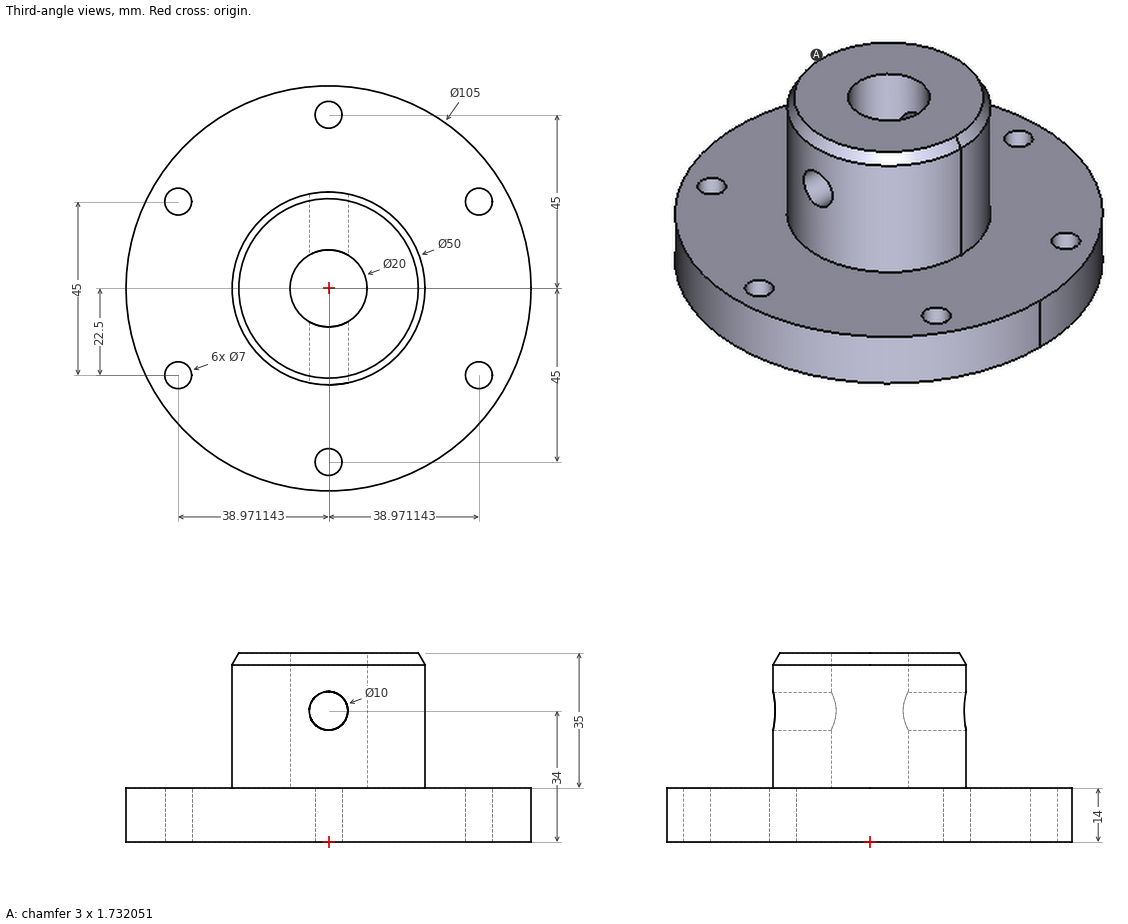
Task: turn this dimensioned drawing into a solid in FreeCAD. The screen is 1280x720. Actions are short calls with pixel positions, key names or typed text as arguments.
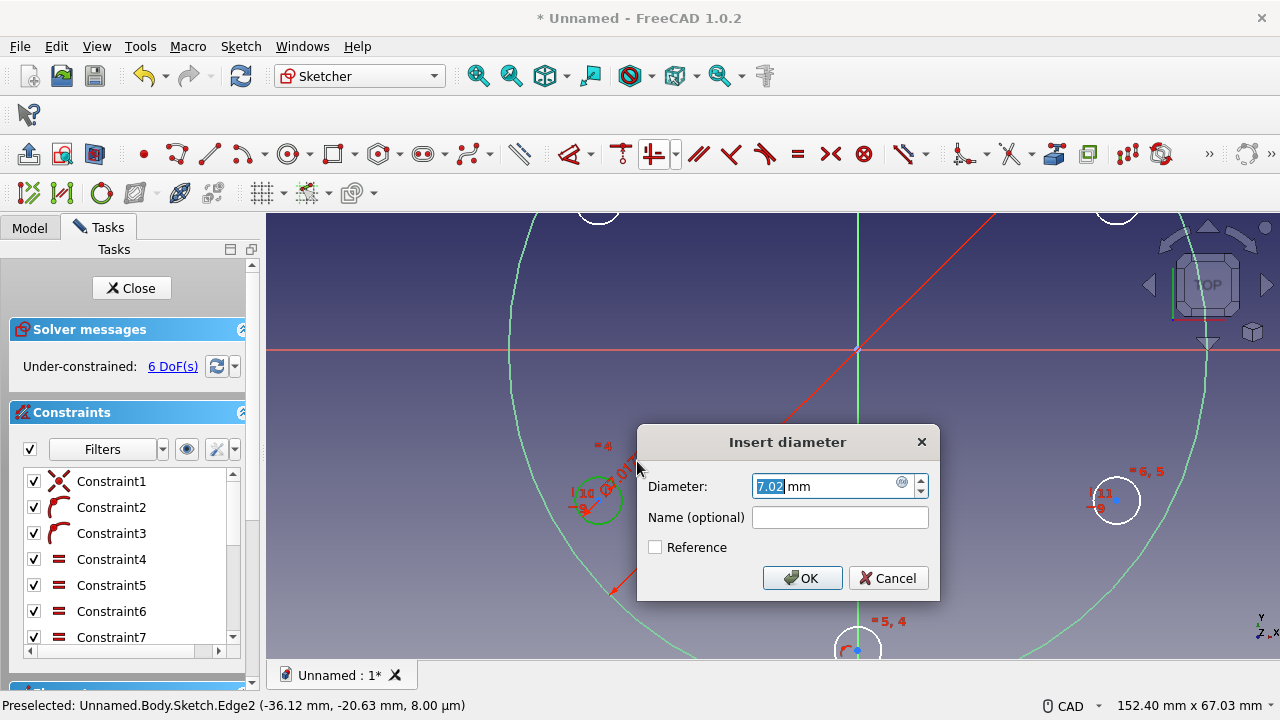
text(7)
key(Return)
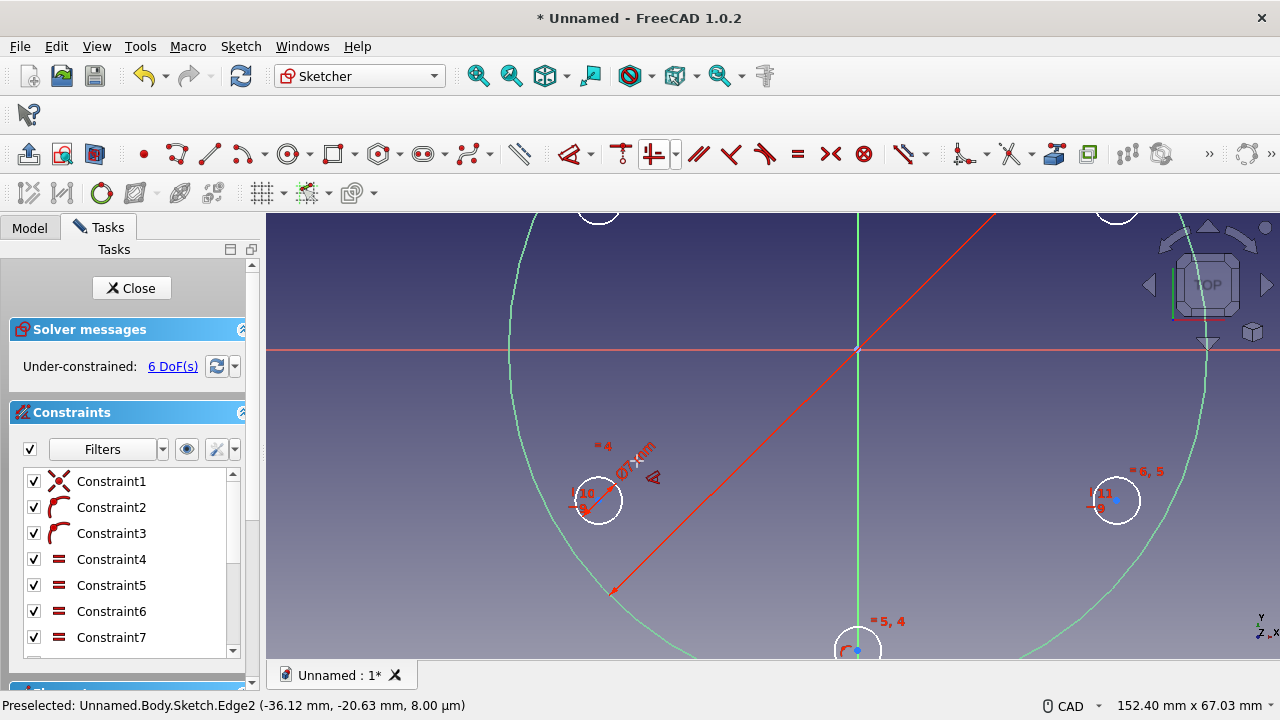
scroll(615, 486, down, 5)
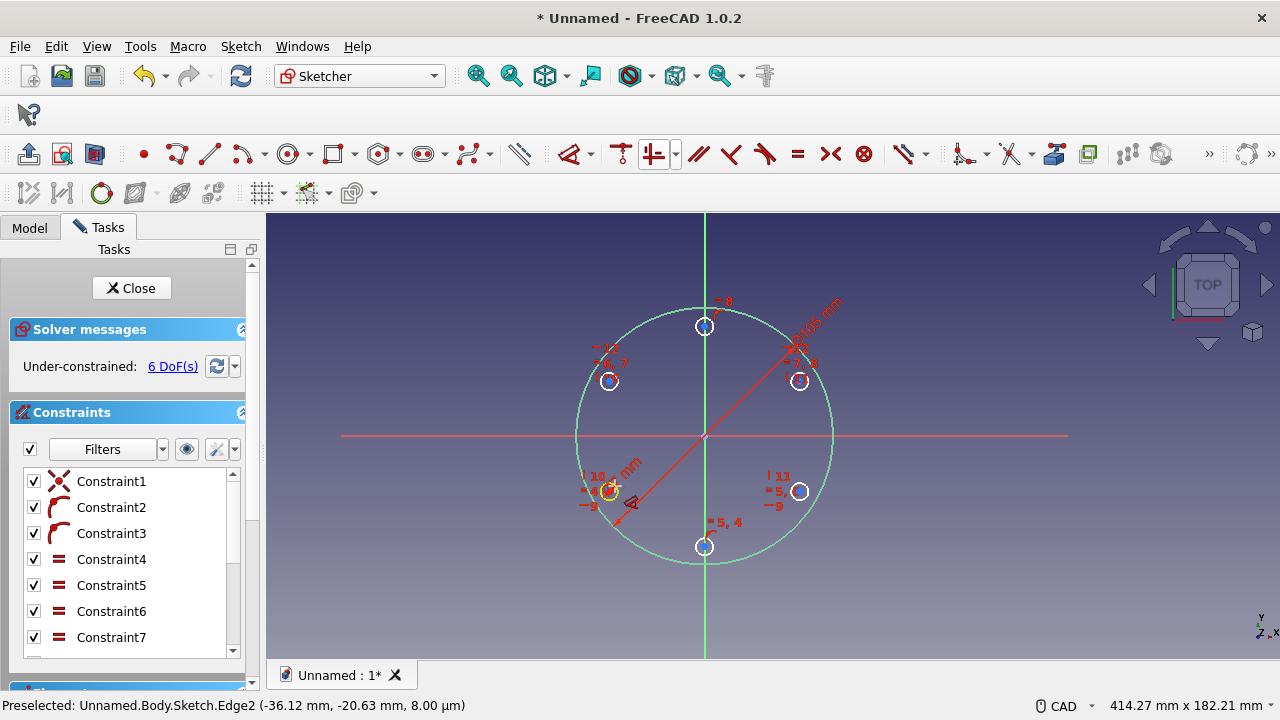
click(705, 547)
click(739, 492)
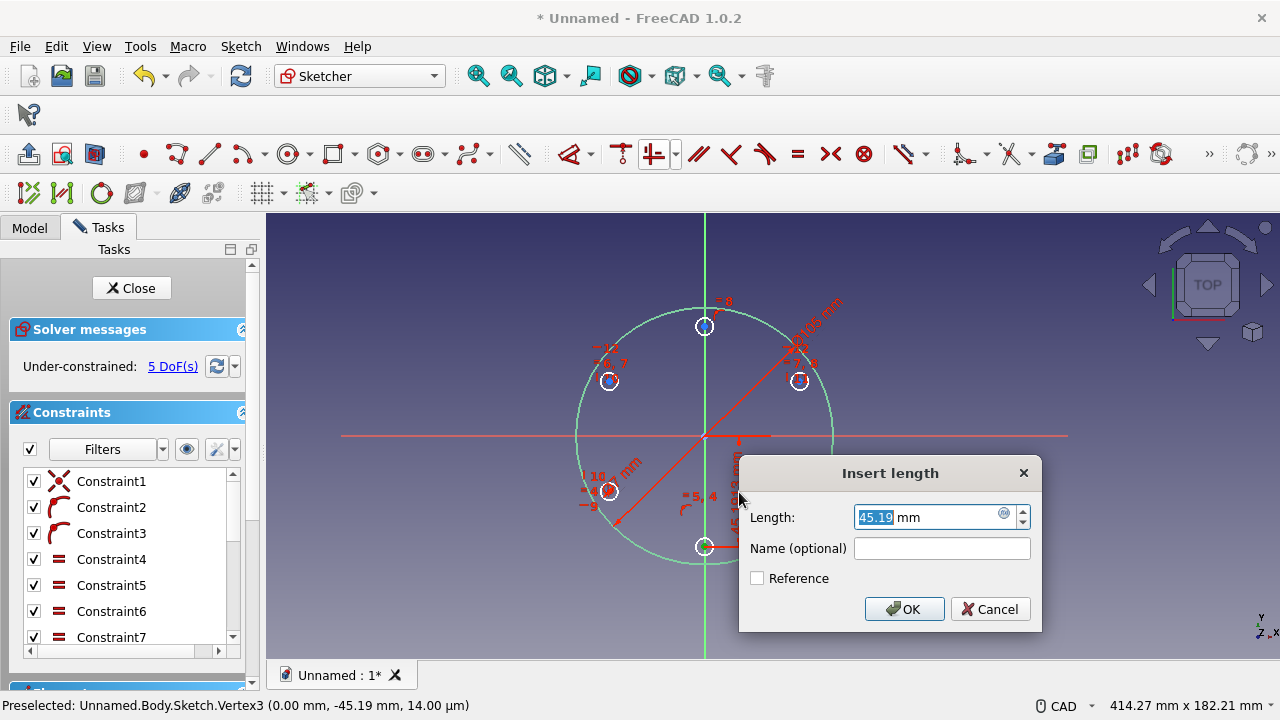
text(45)
key(Return)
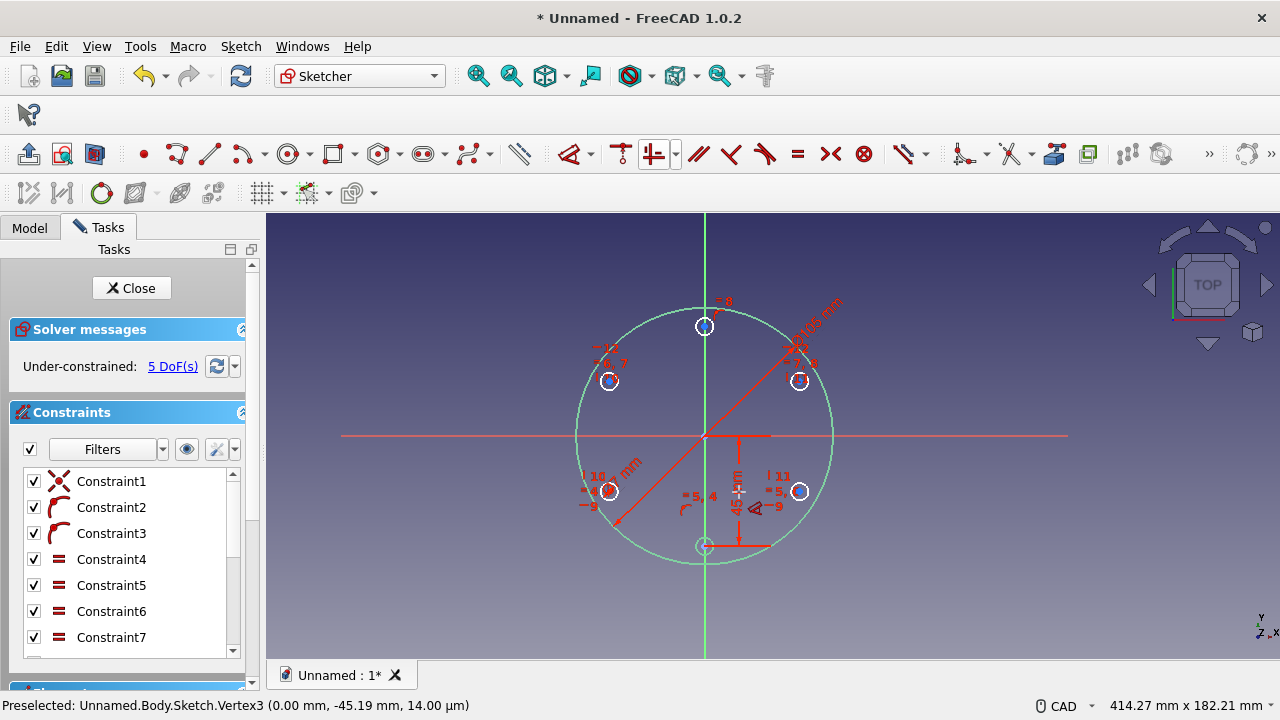
click(705, 327)
click(739, 381)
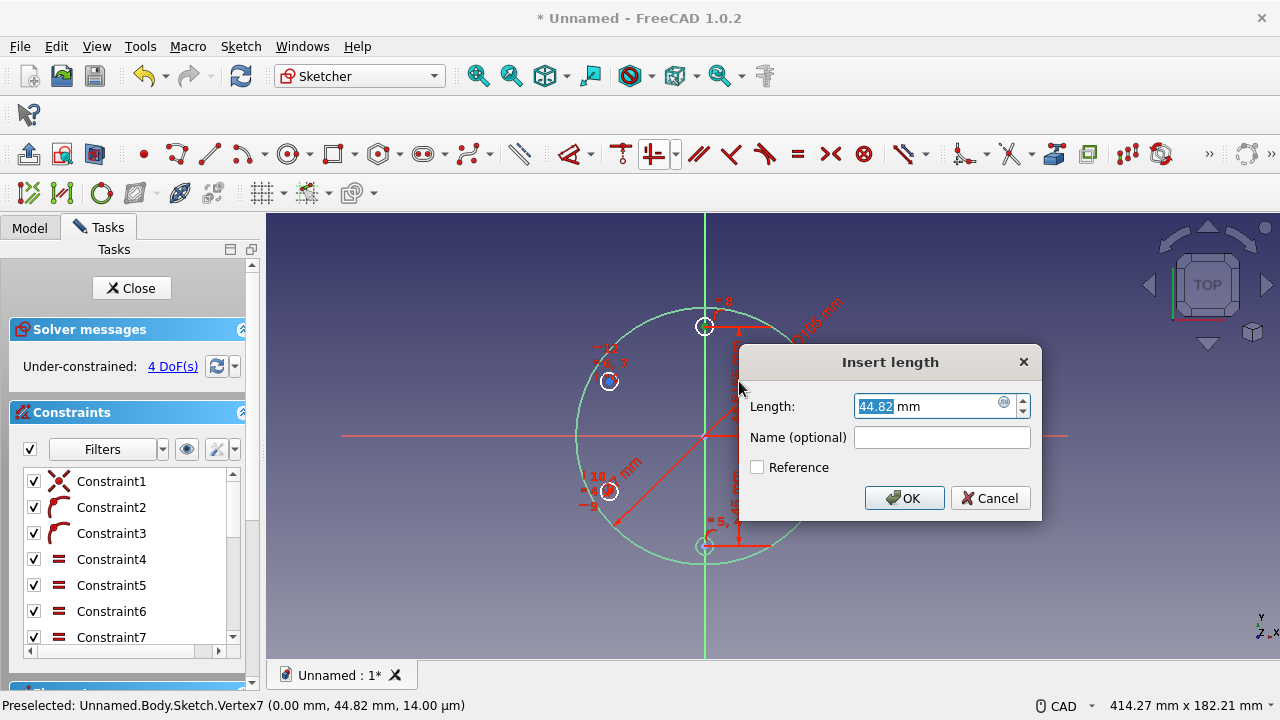
text(45)
key(Return)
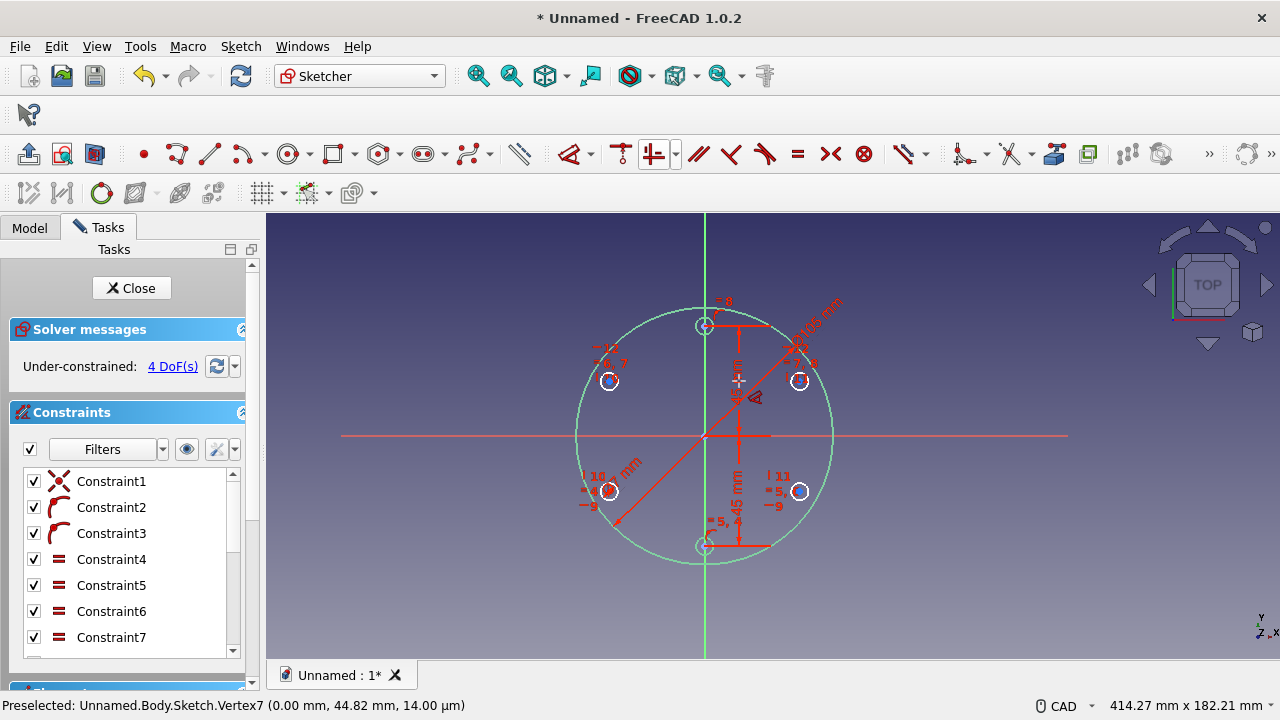
click(609, 492)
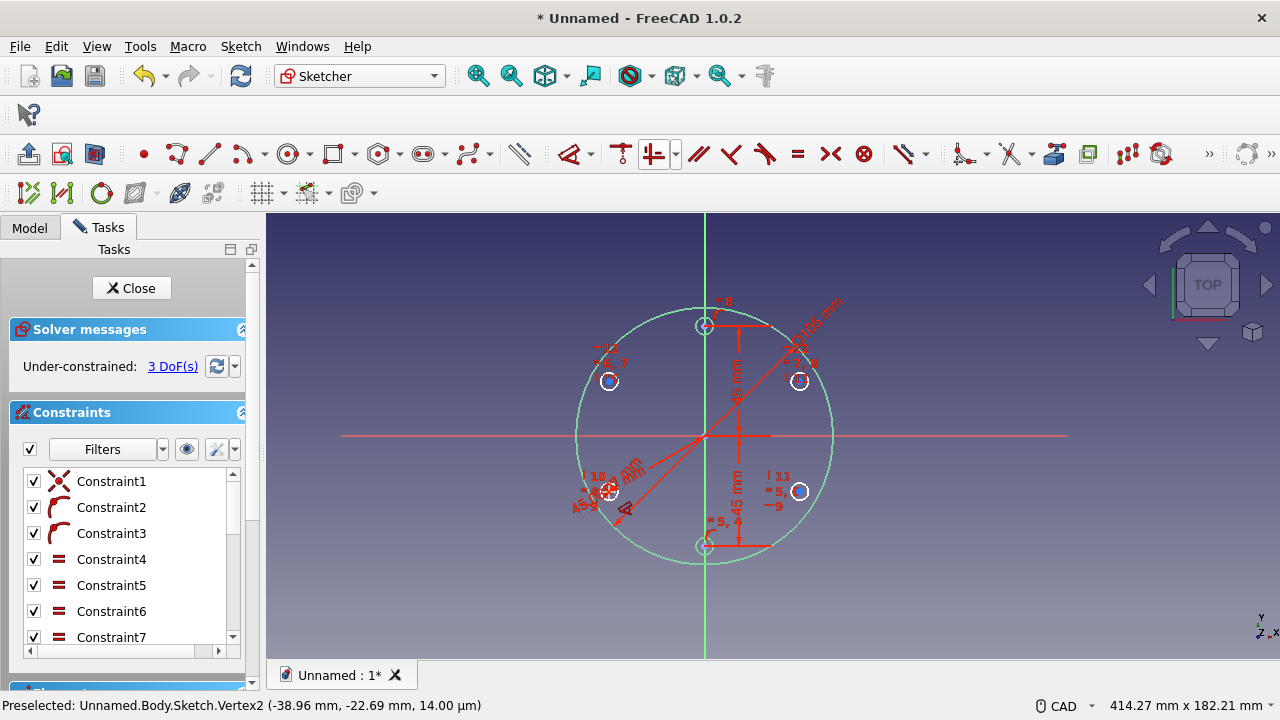
click(609, 382)
click(643, 411)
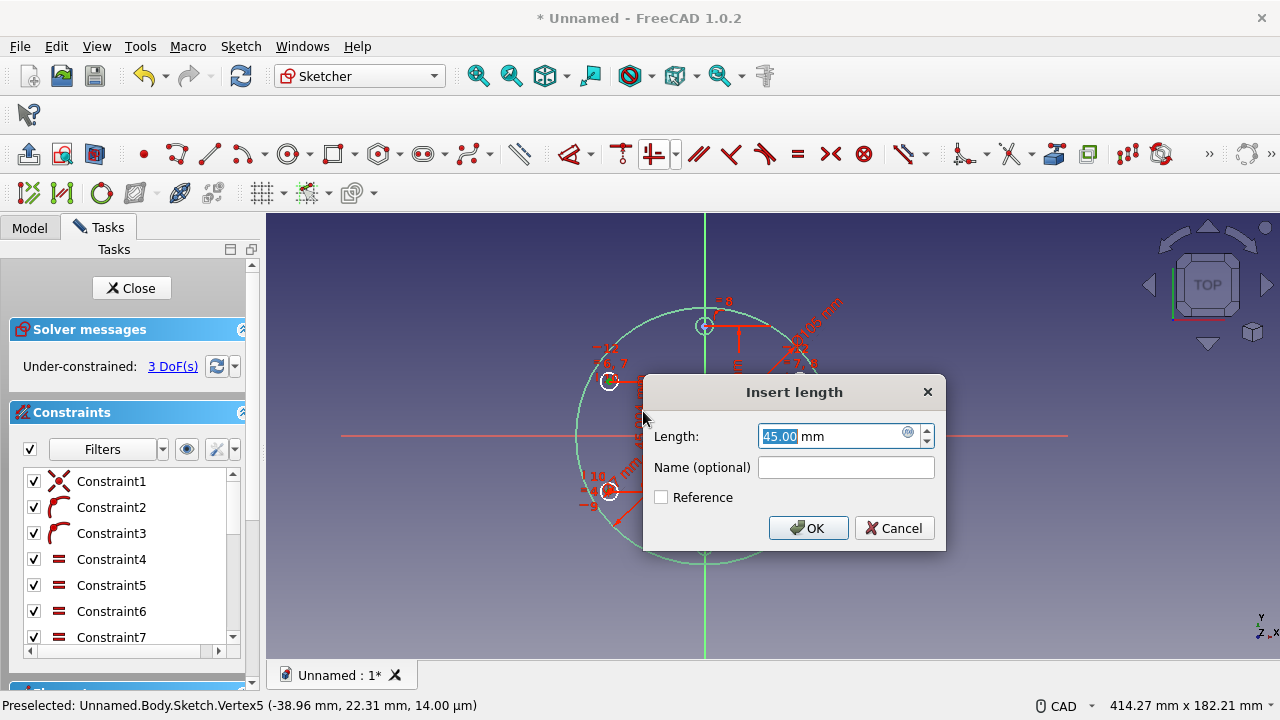
text(45)
key(Return)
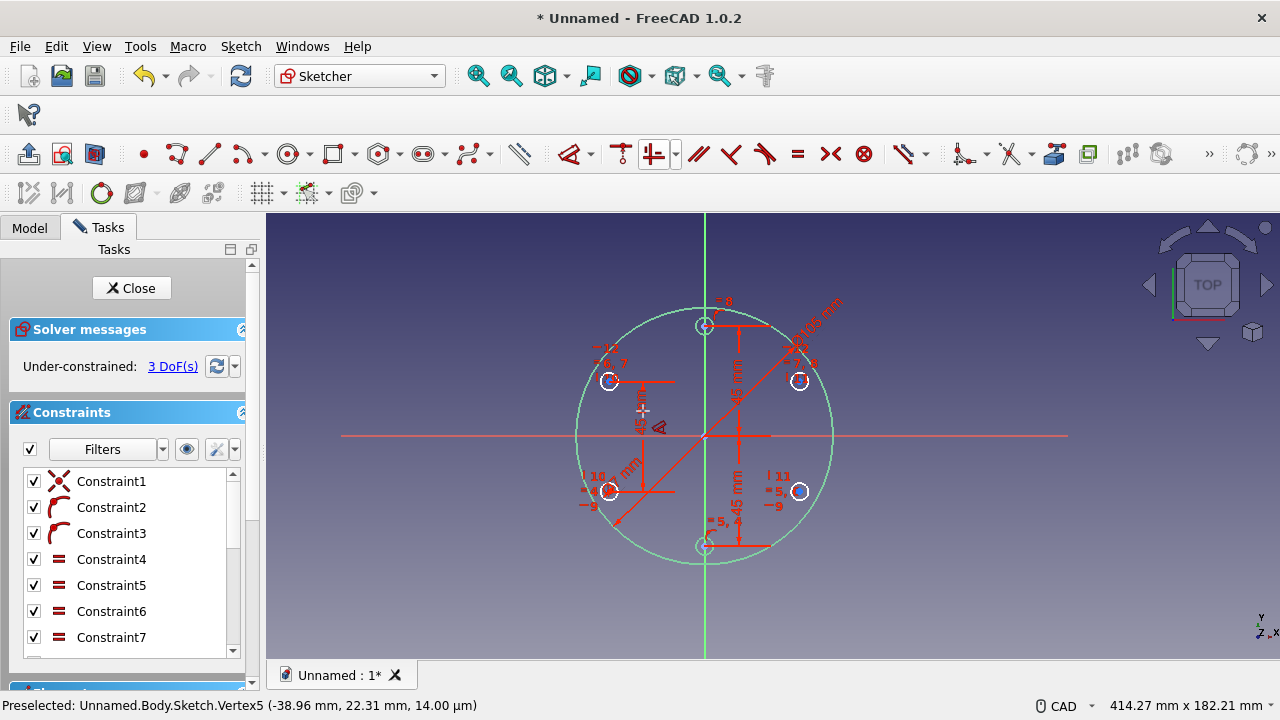
click(609, 492)
click(739, 464)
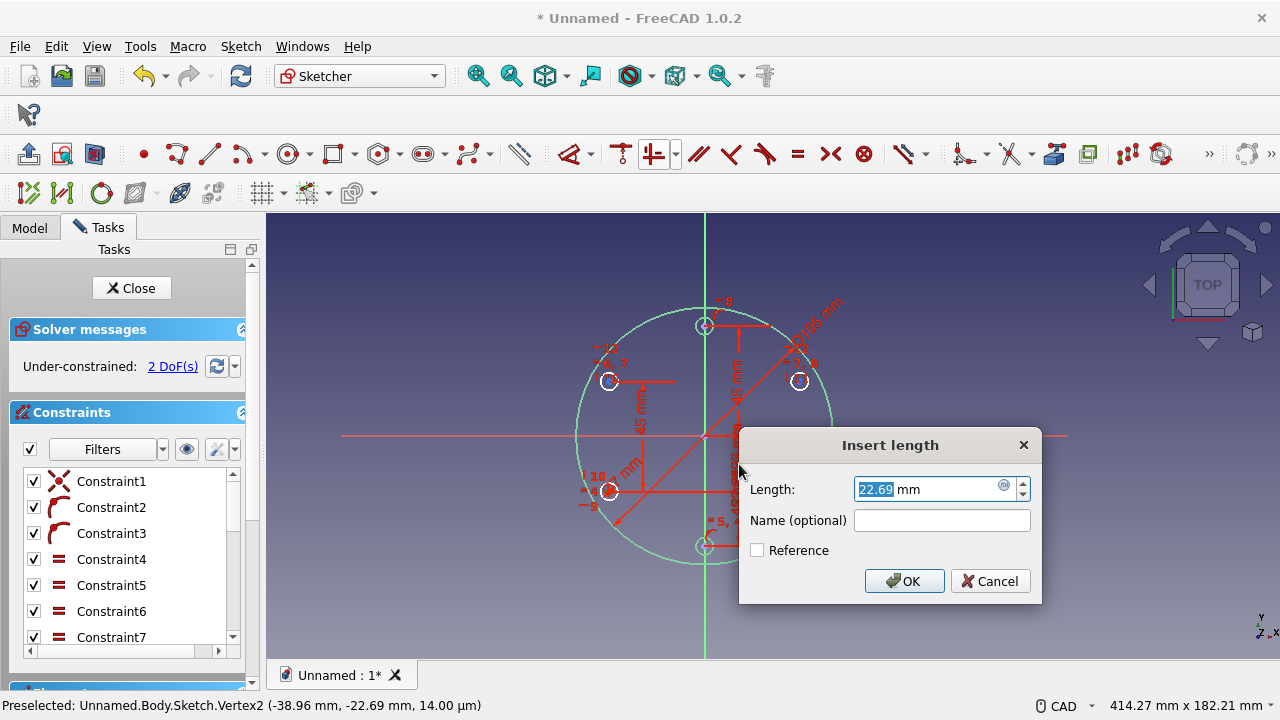
text(22.5)
key(Return)